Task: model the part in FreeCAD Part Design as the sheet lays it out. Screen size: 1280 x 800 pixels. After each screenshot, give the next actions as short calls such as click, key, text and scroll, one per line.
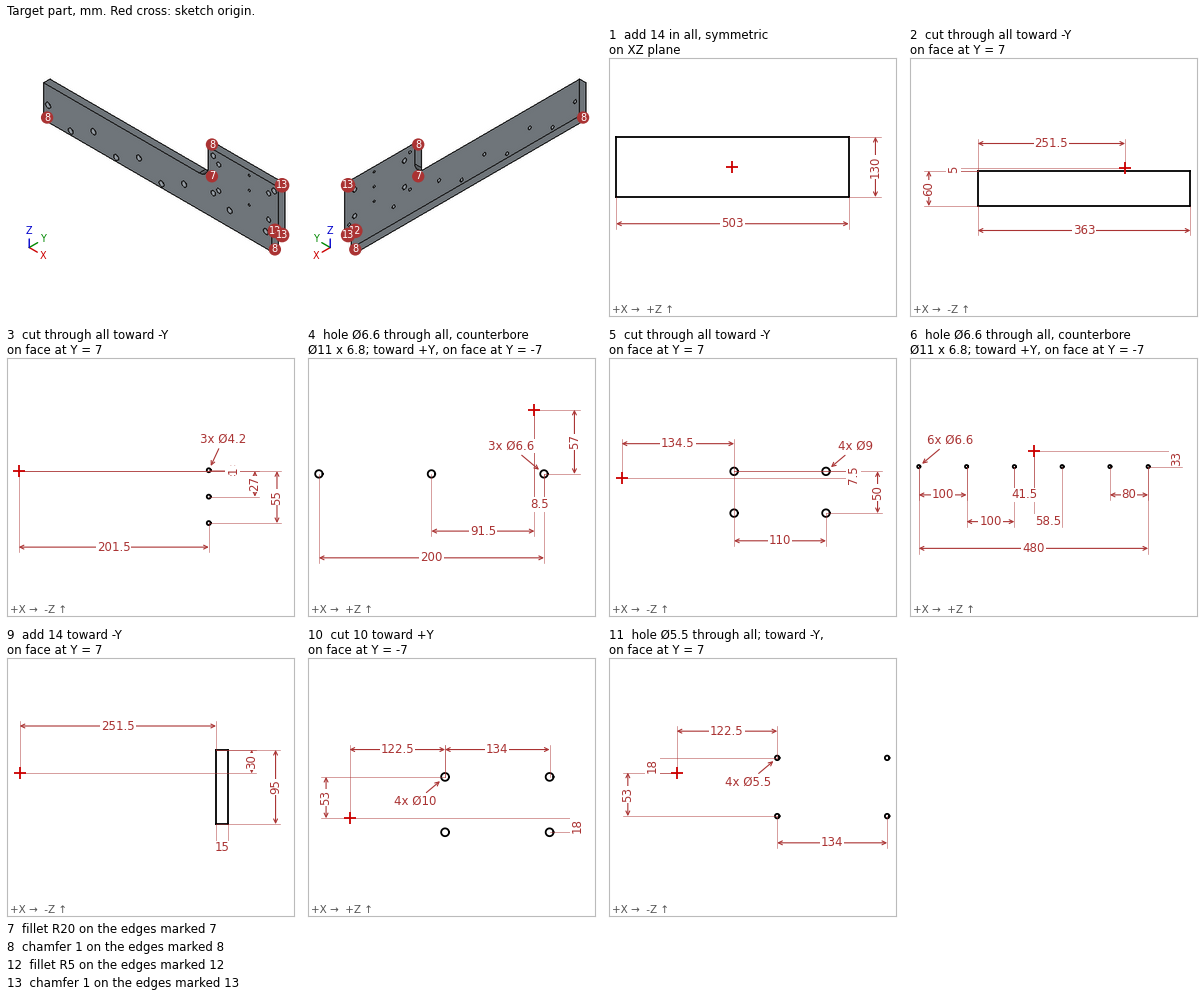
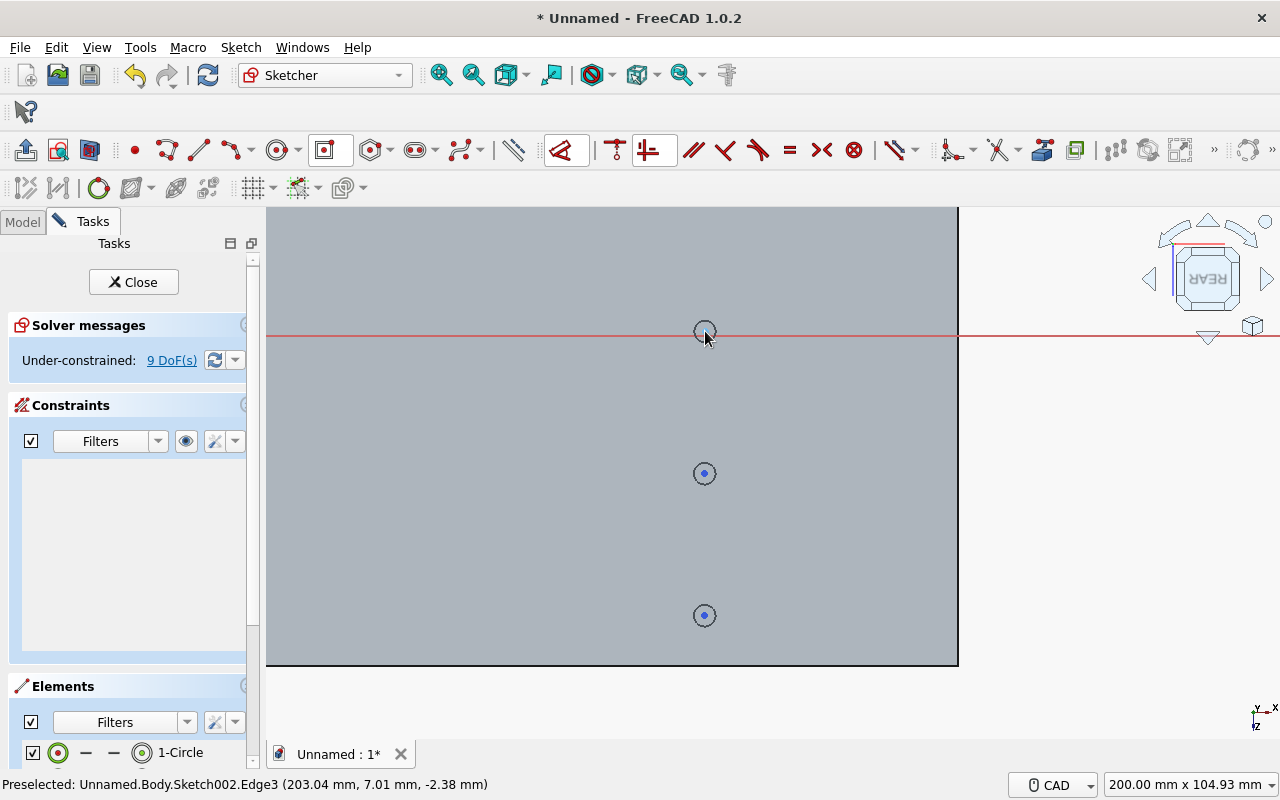
scroll(712, 608, up, 2)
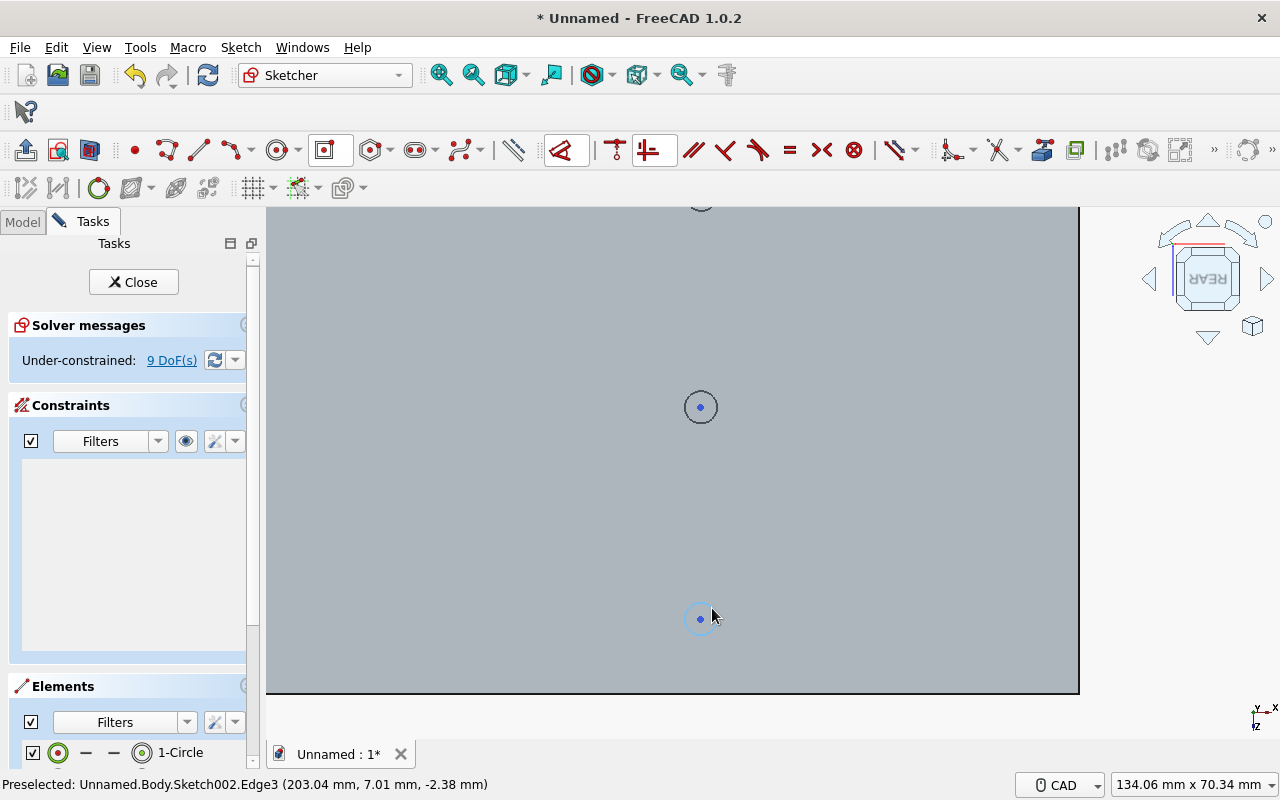
click(712, 608)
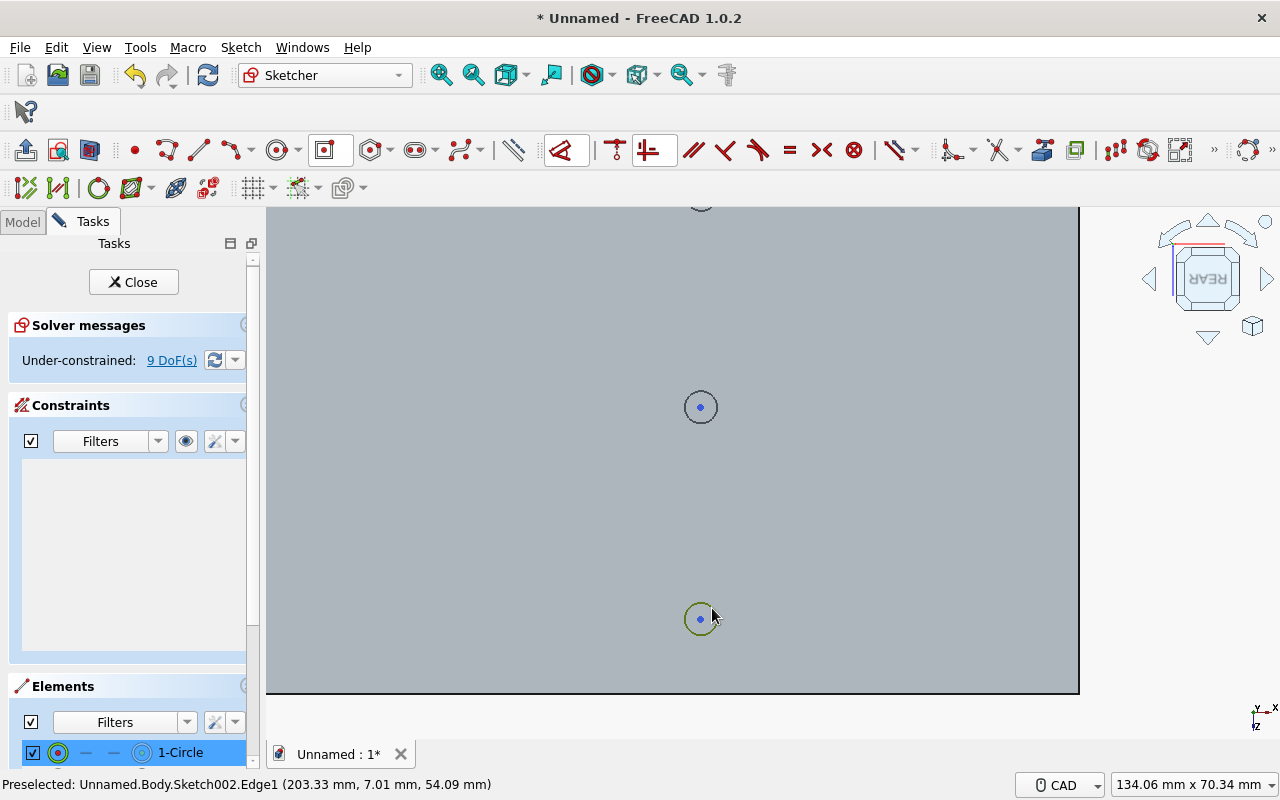
click(712, 396)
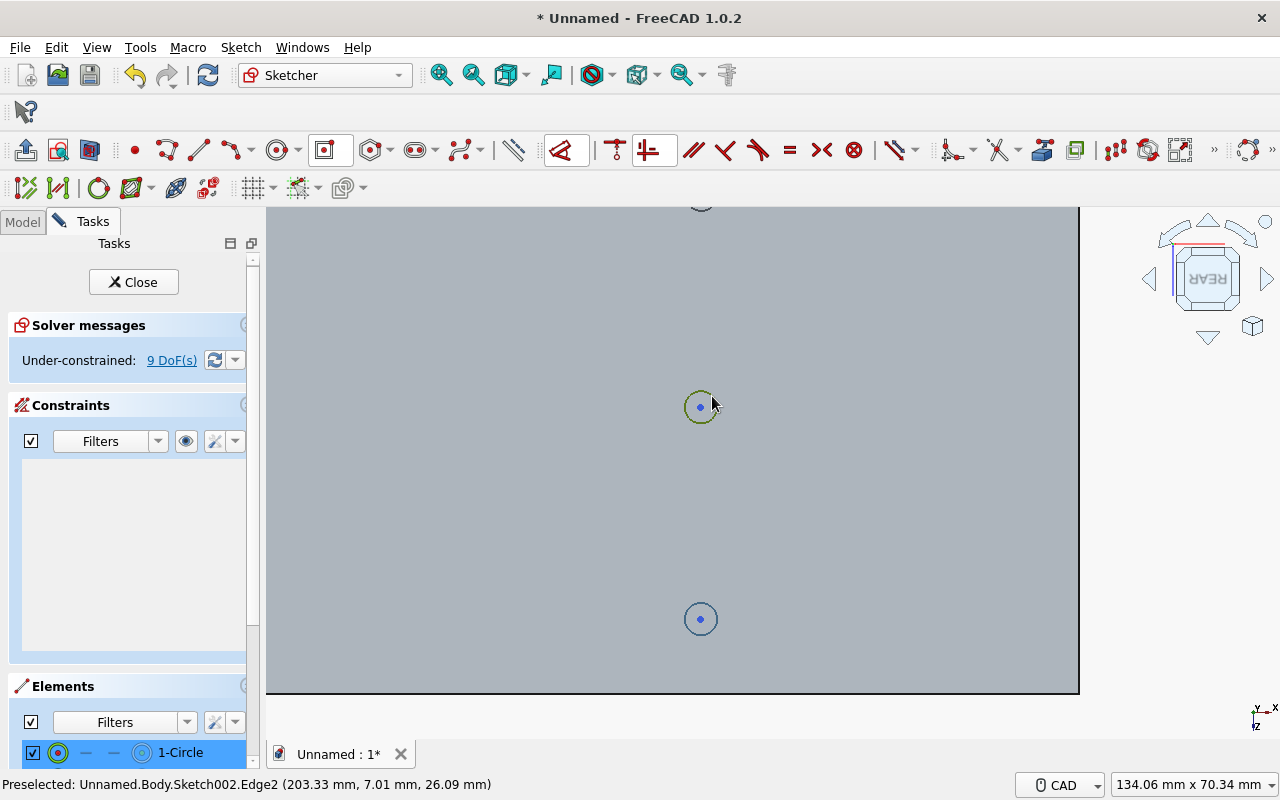
scroll(711, 608, down, 2)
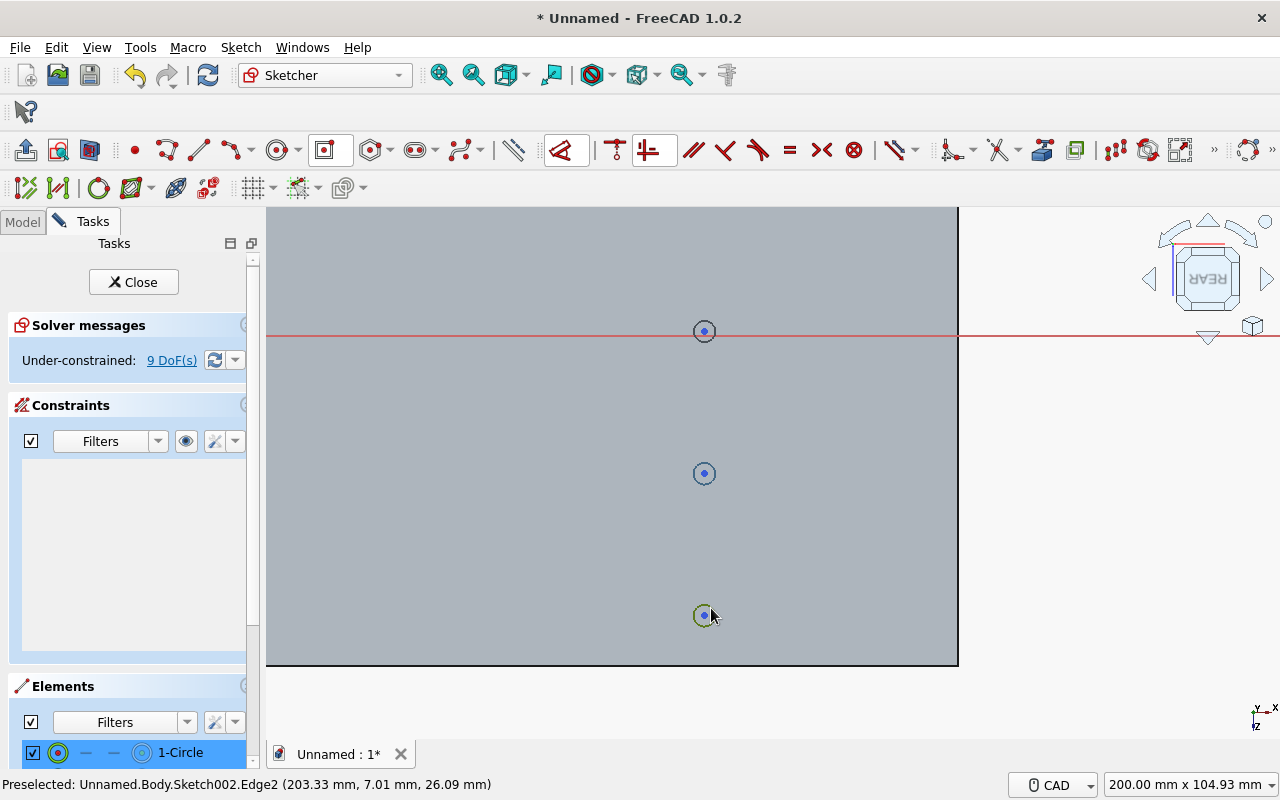
scroll(712, 324, up, 2)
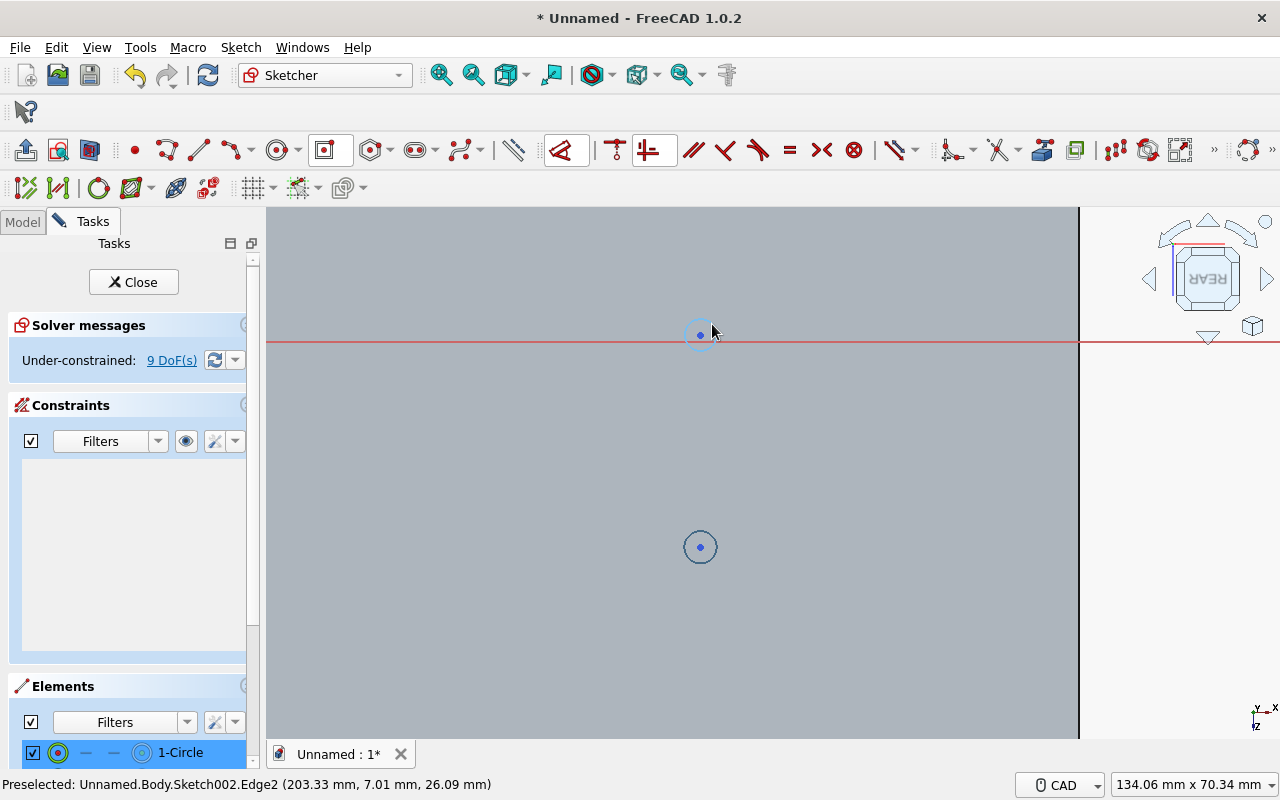
click(712, 324)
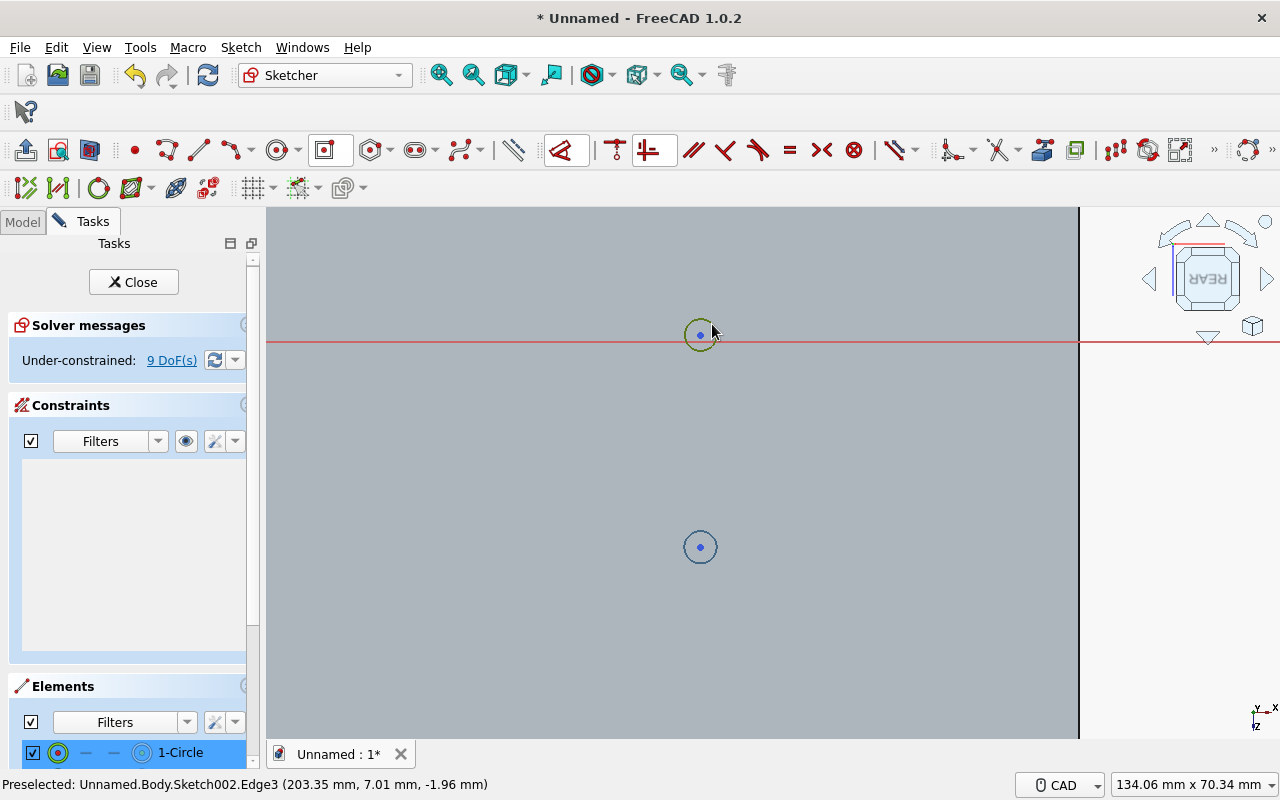
click(790, 150)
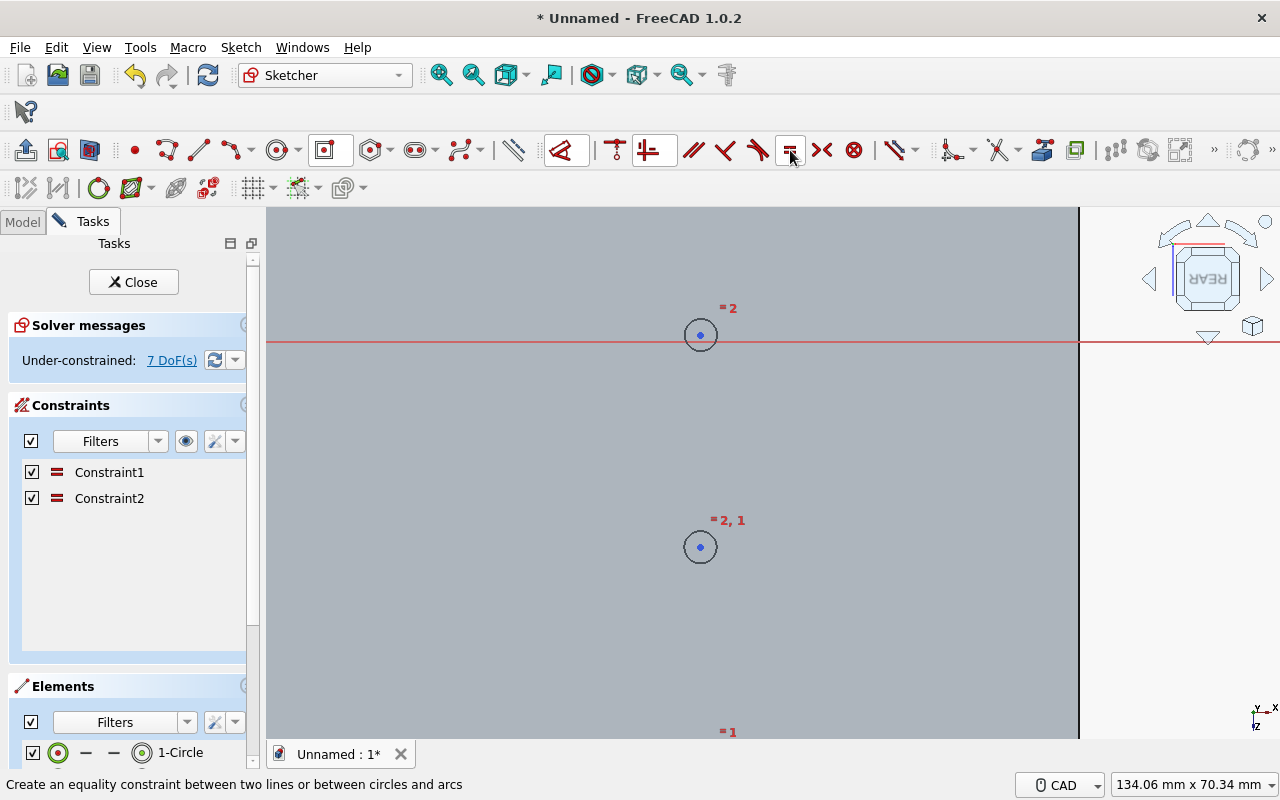
scroll(712, 324, down, 2)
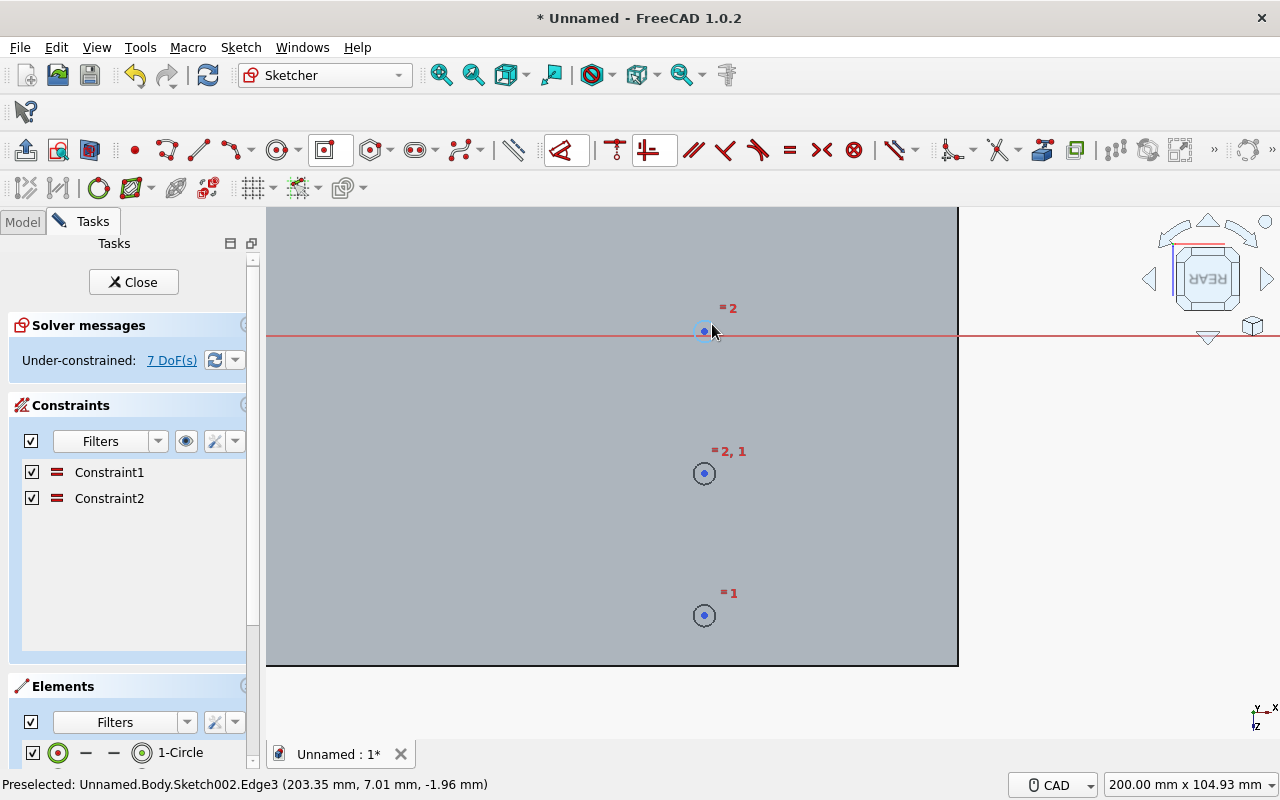
click(704, 616)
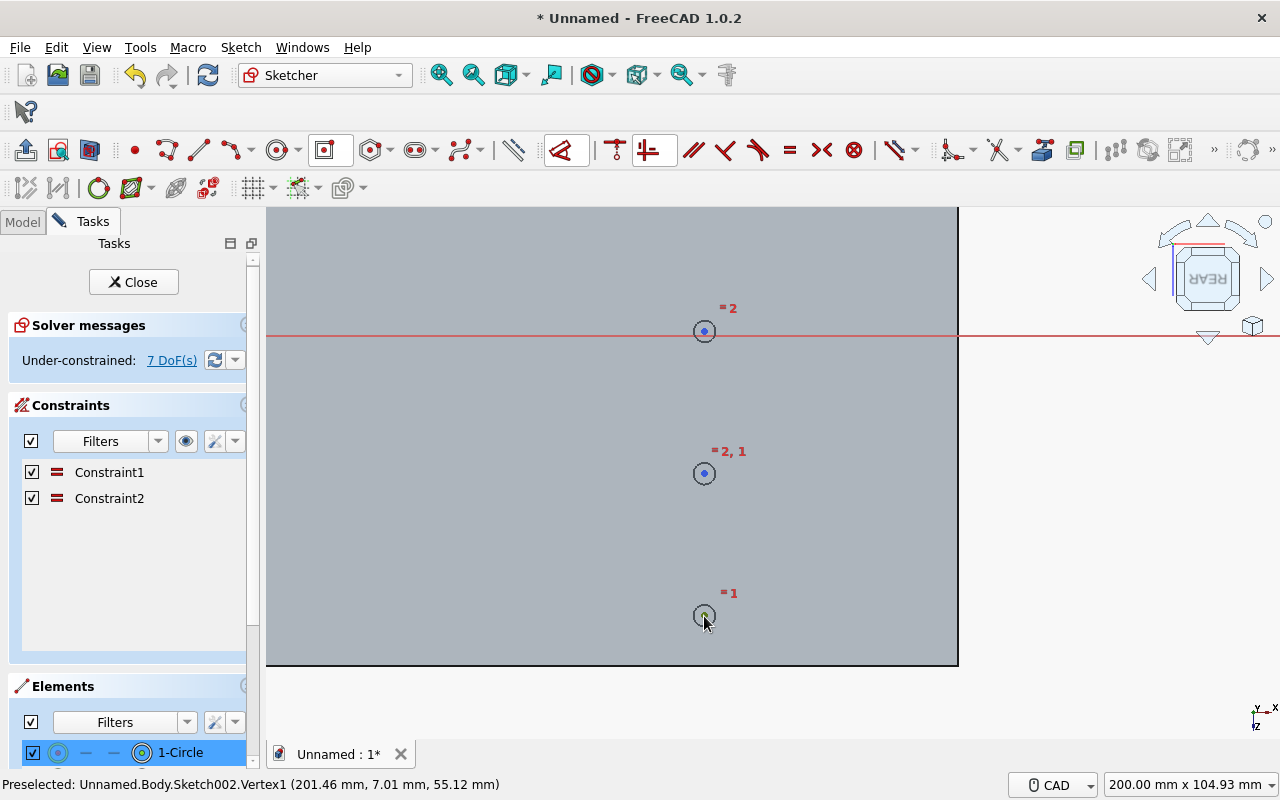
click(704, 474)